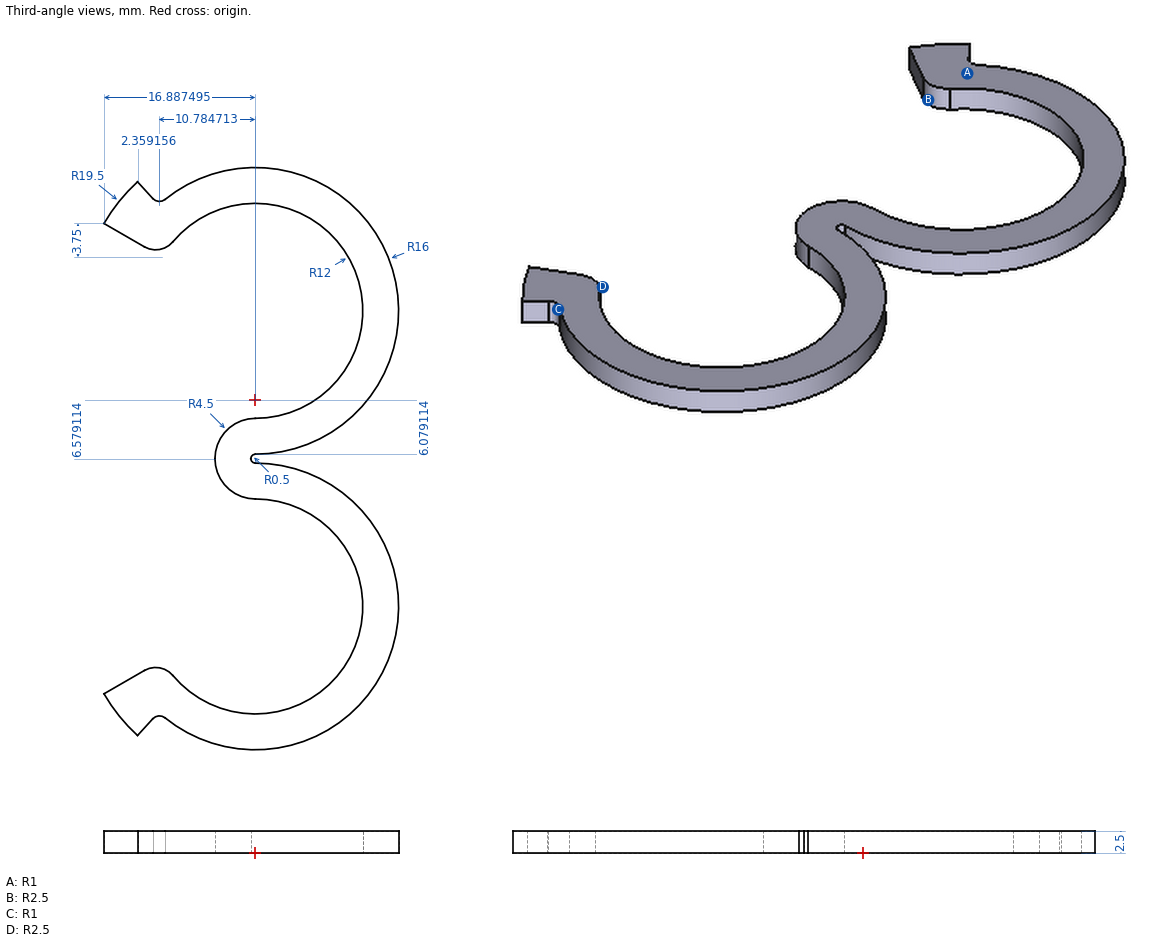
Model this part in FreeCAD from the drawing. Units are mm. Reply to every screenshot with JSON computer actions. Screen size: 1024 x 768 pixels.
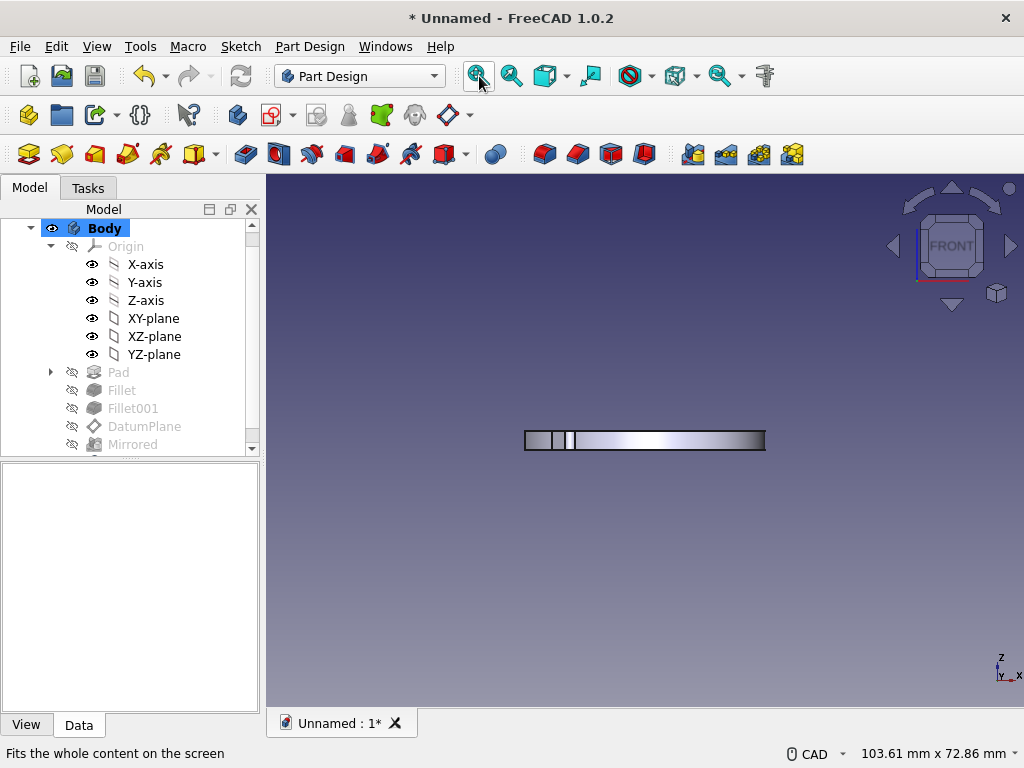
{"action": "scroll", "coordinate": [572, 440], "scroll_direction": "up", "scroll_amount": 4}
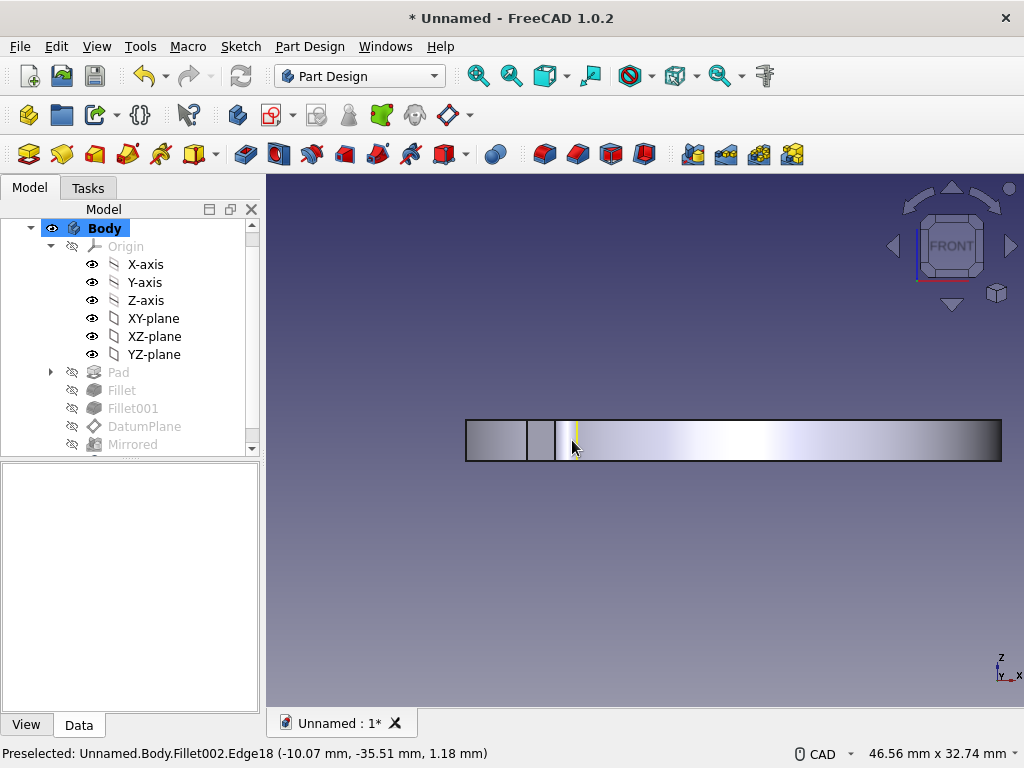
{"action": "left_click", "coordinate": [479, 76]}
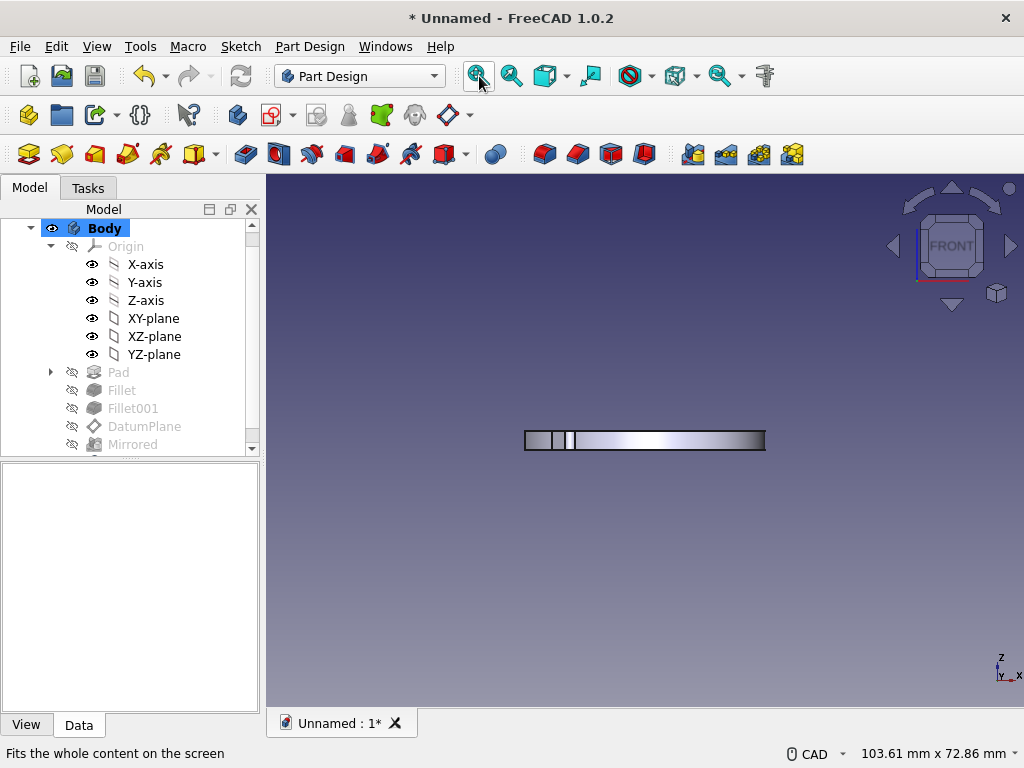
{"action": "key", "text": "3"}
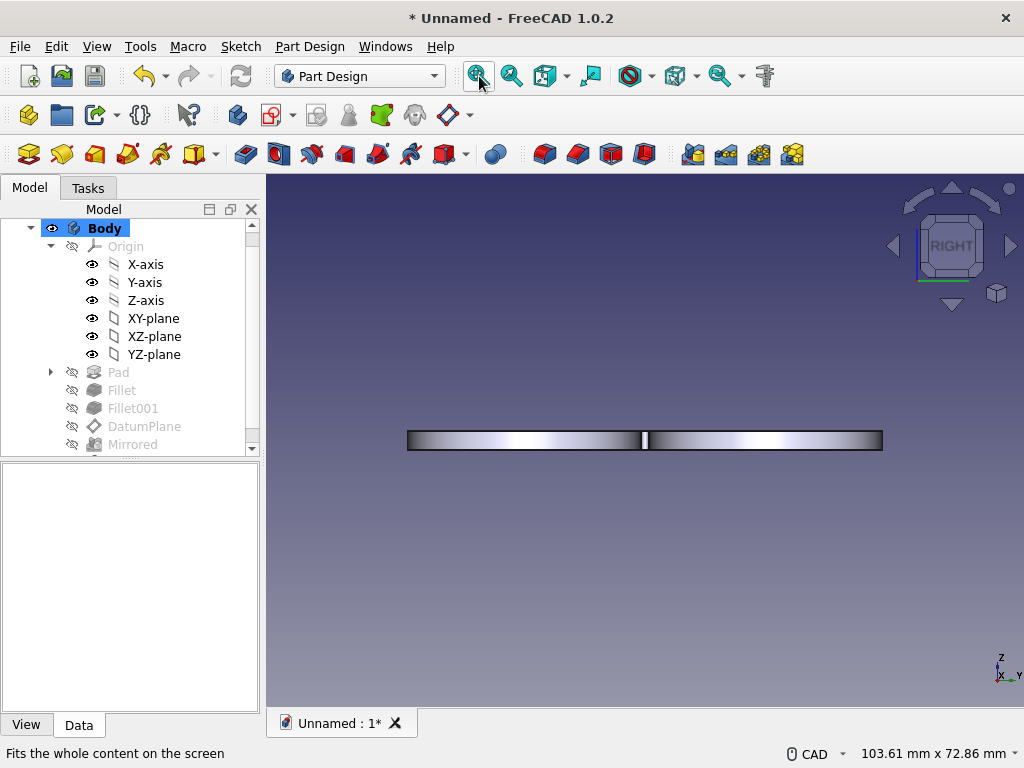
{"action": "scroll", "coordinate": [480, 439], "scroll_direction": "up", "scroll_amount": 4}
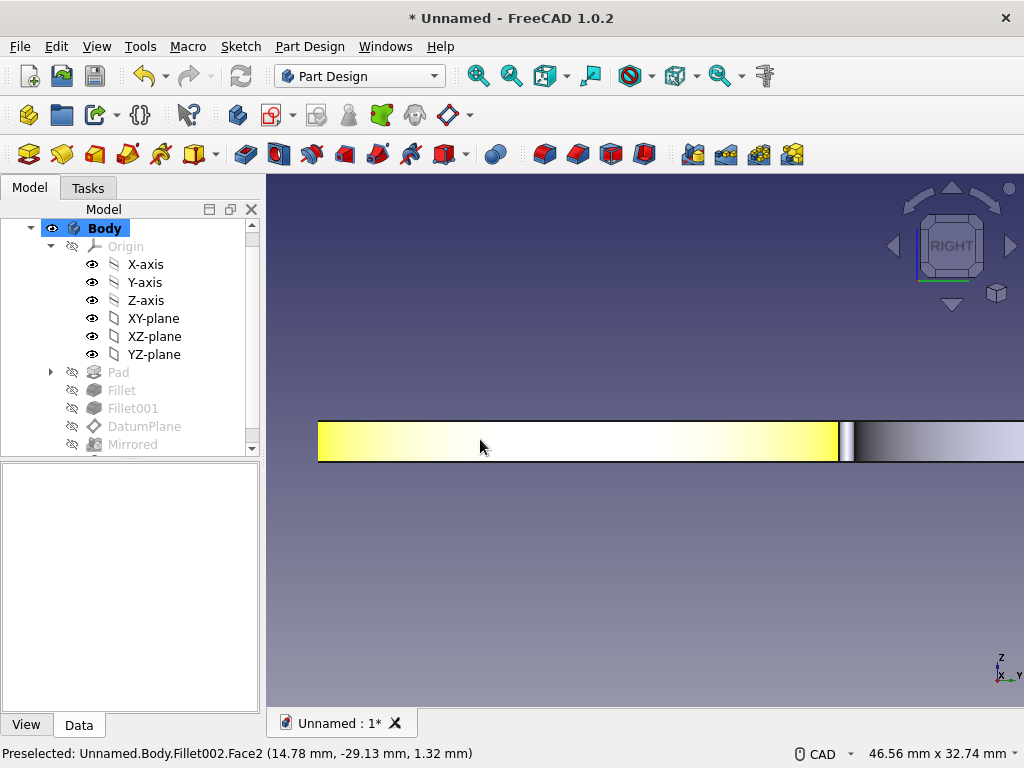
{"action": "left_click", "coordinate": [479, 76]}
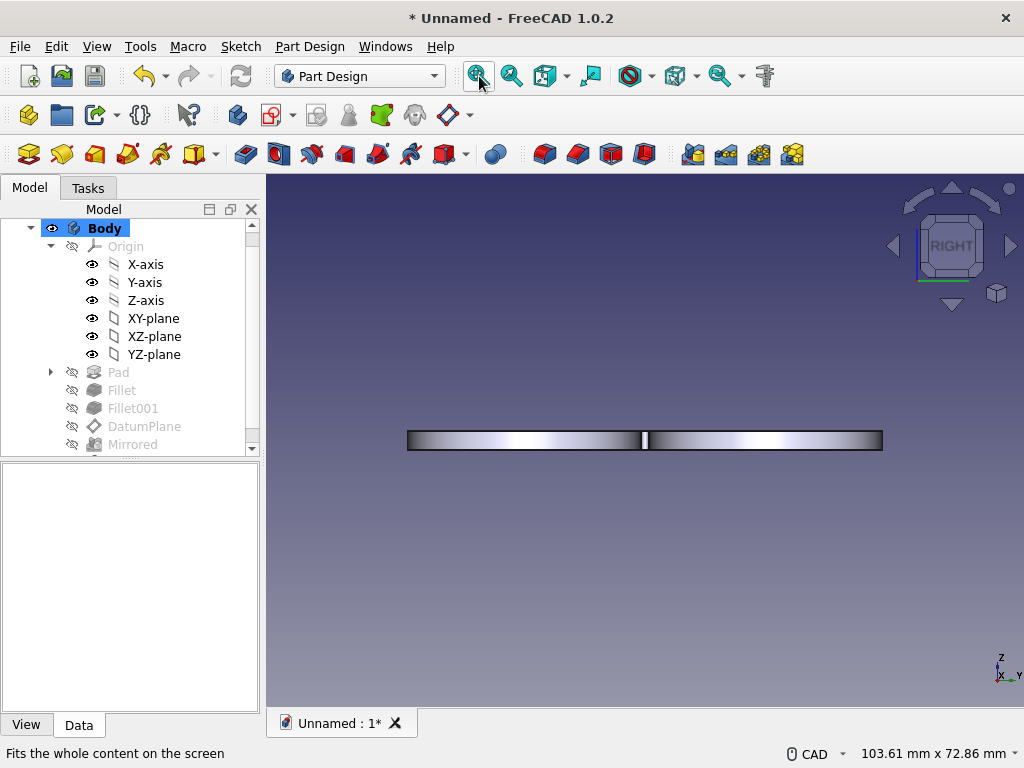
{"action": "key", "text": "5"}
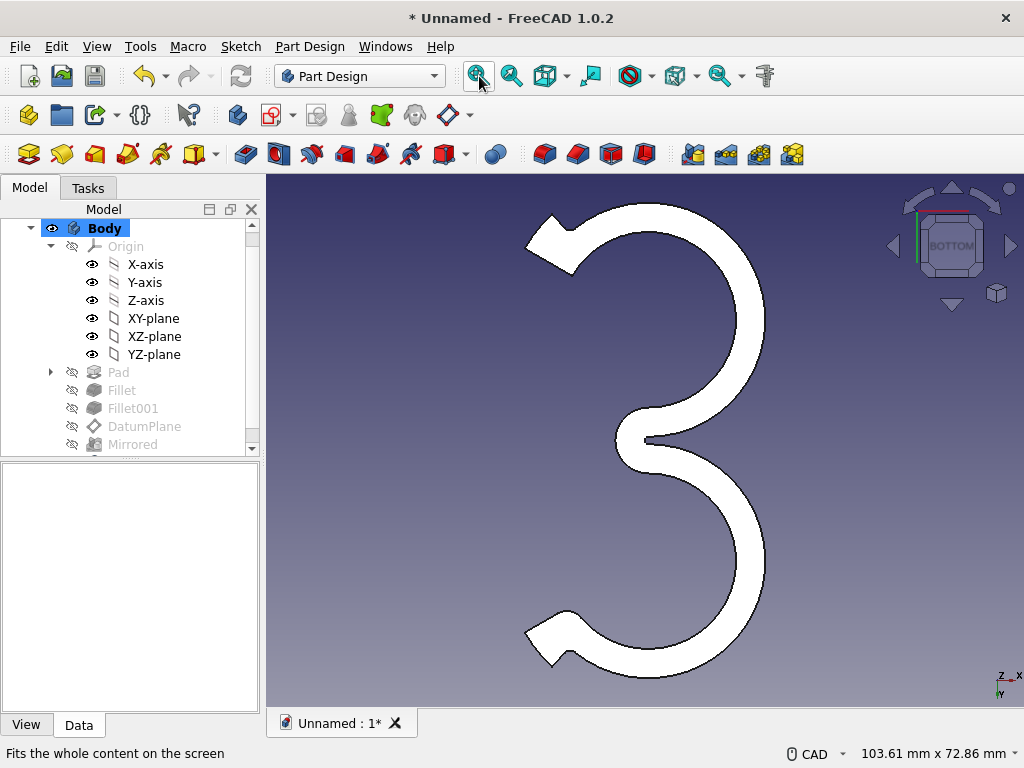
{"action": "scroll", "coordinate": [572, 275], "scroll_direction": "up", "scroll_amount": 4}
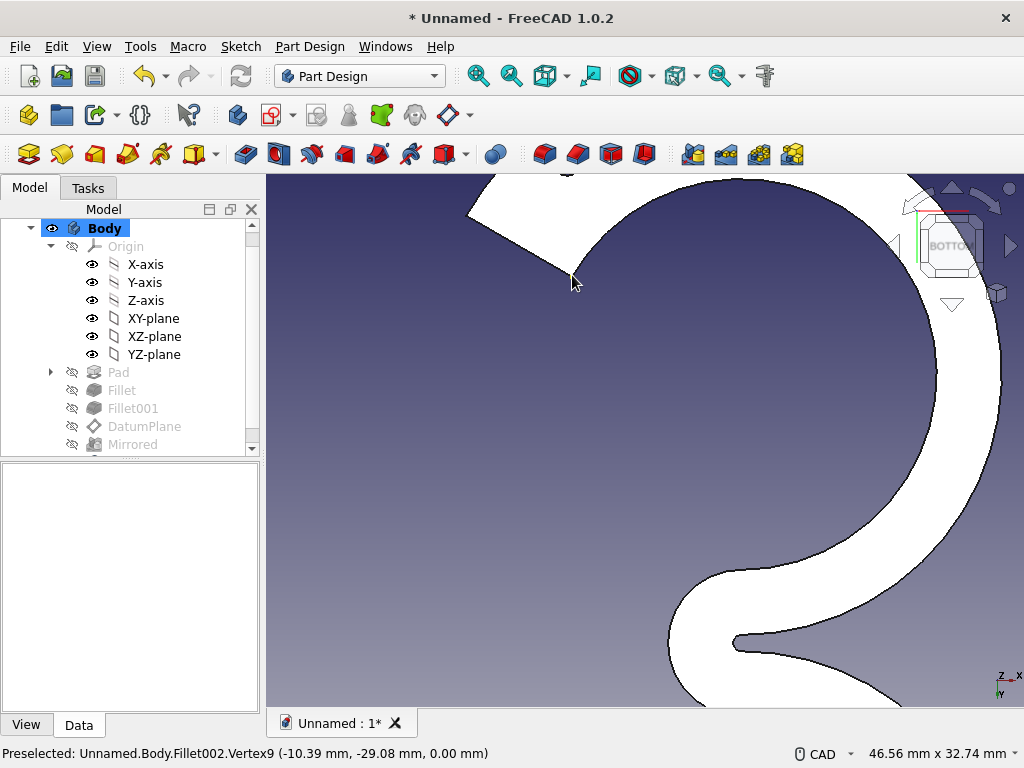
{"action": "left_click", "coordinate": [479, 76]}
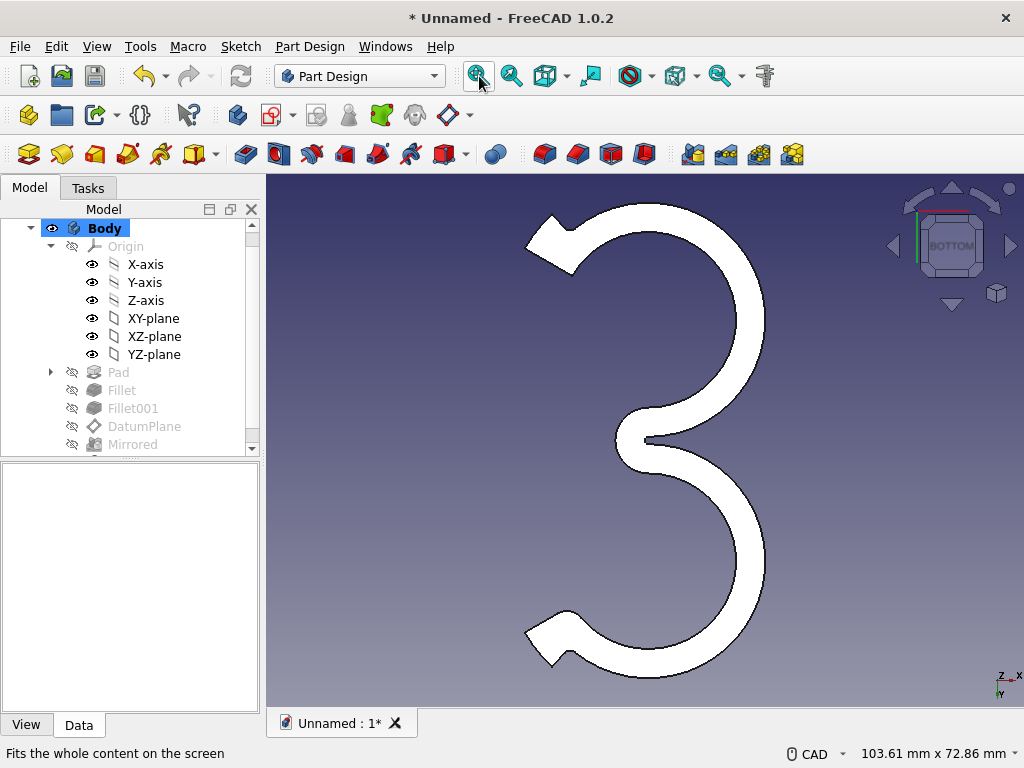
{"action": "key", "text": "4"}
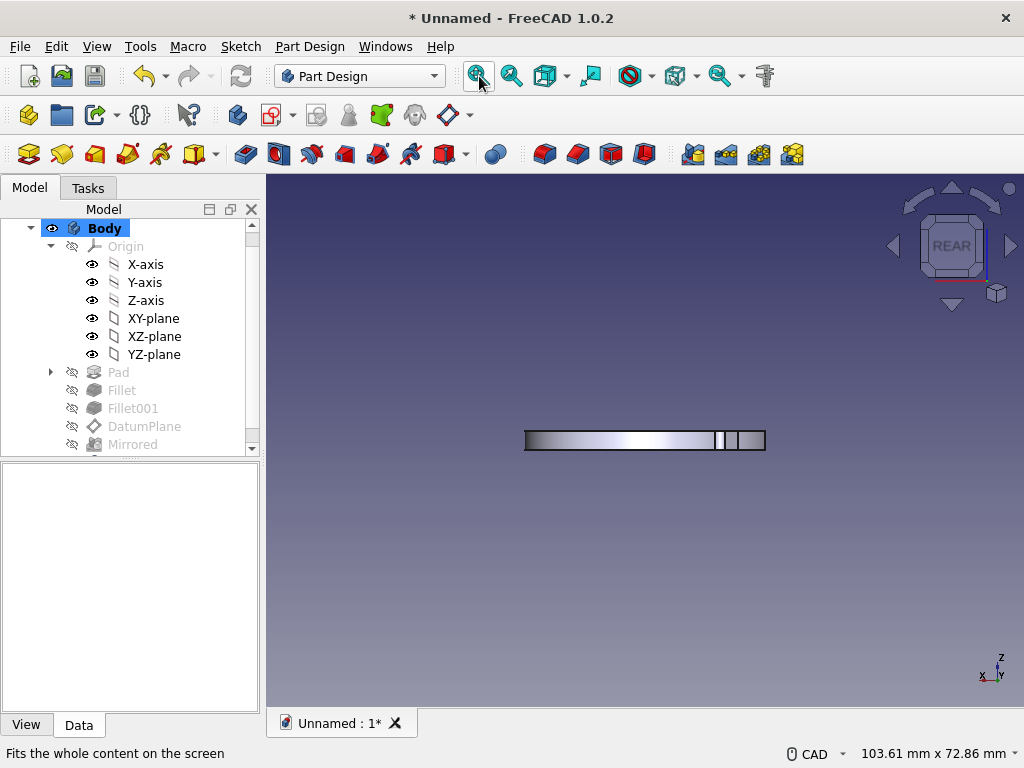
{"action": "left_click", "coordinate": [479, 76]}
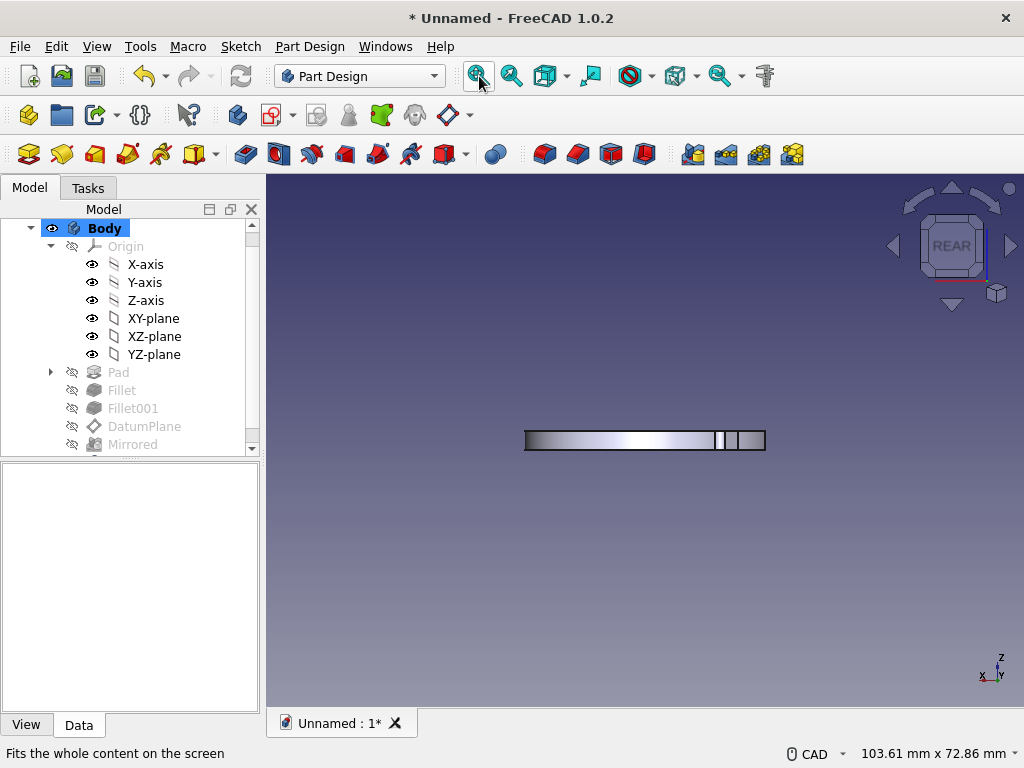
{"action": "scroll", "coordinate": [718, 440], "scroll_direction": "up", "scroll_amount": 4}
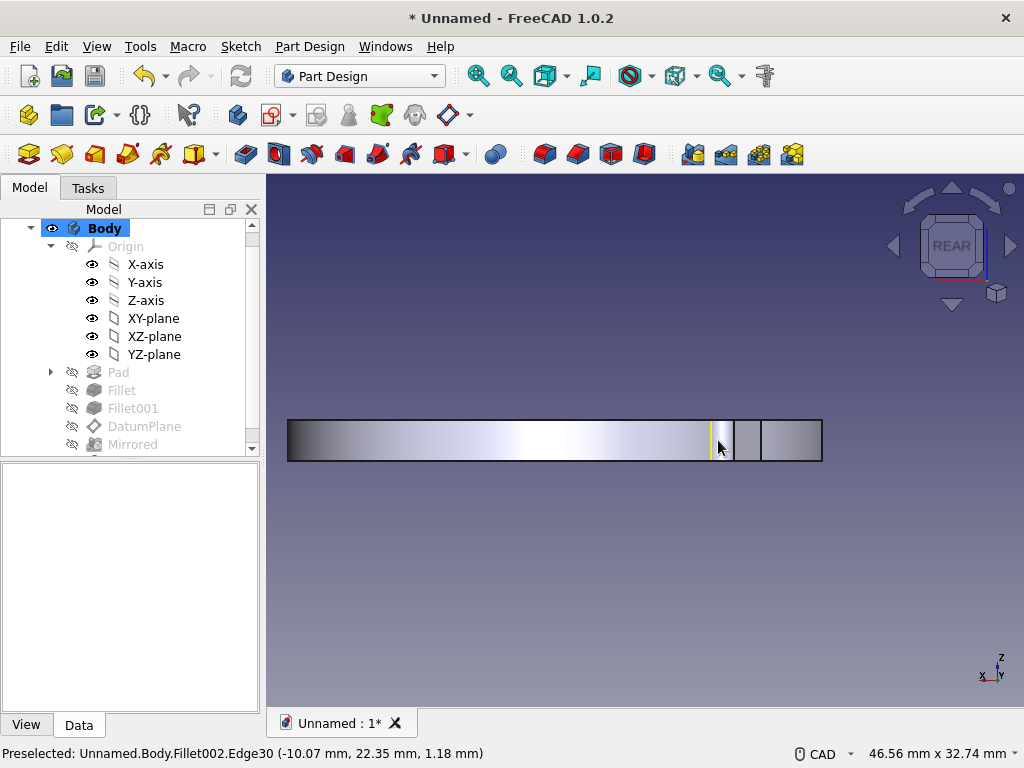
{"action": "left_click", "coordinate": [479, 76]}